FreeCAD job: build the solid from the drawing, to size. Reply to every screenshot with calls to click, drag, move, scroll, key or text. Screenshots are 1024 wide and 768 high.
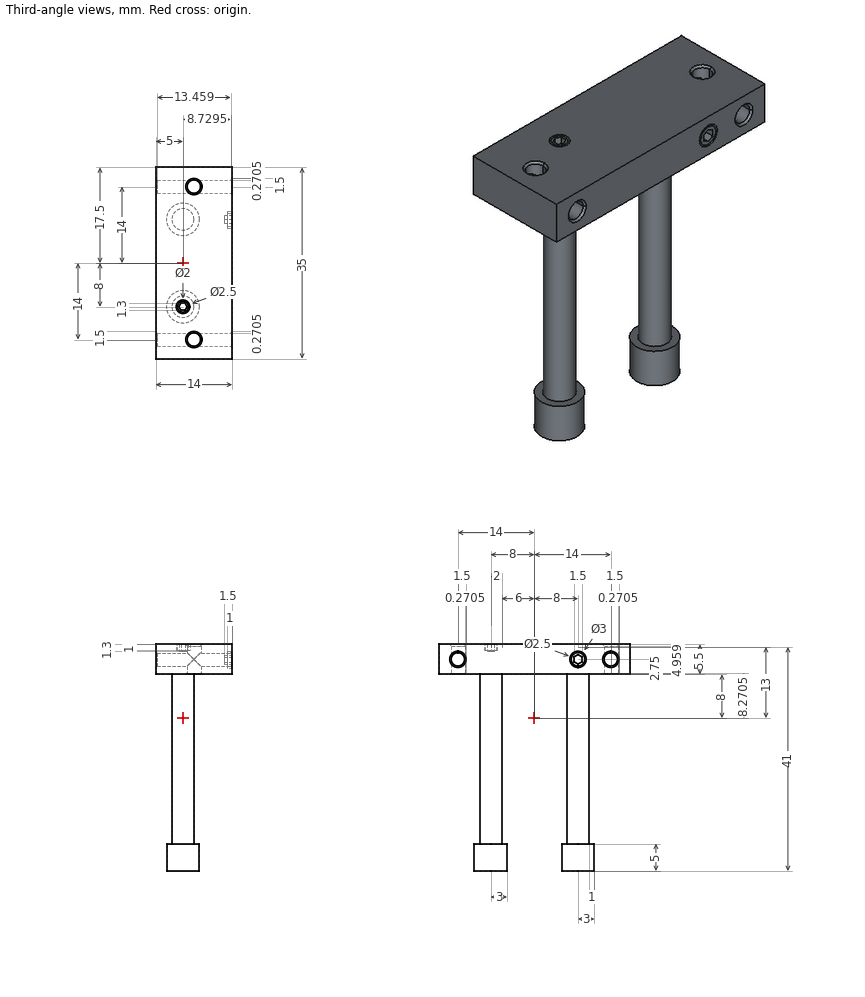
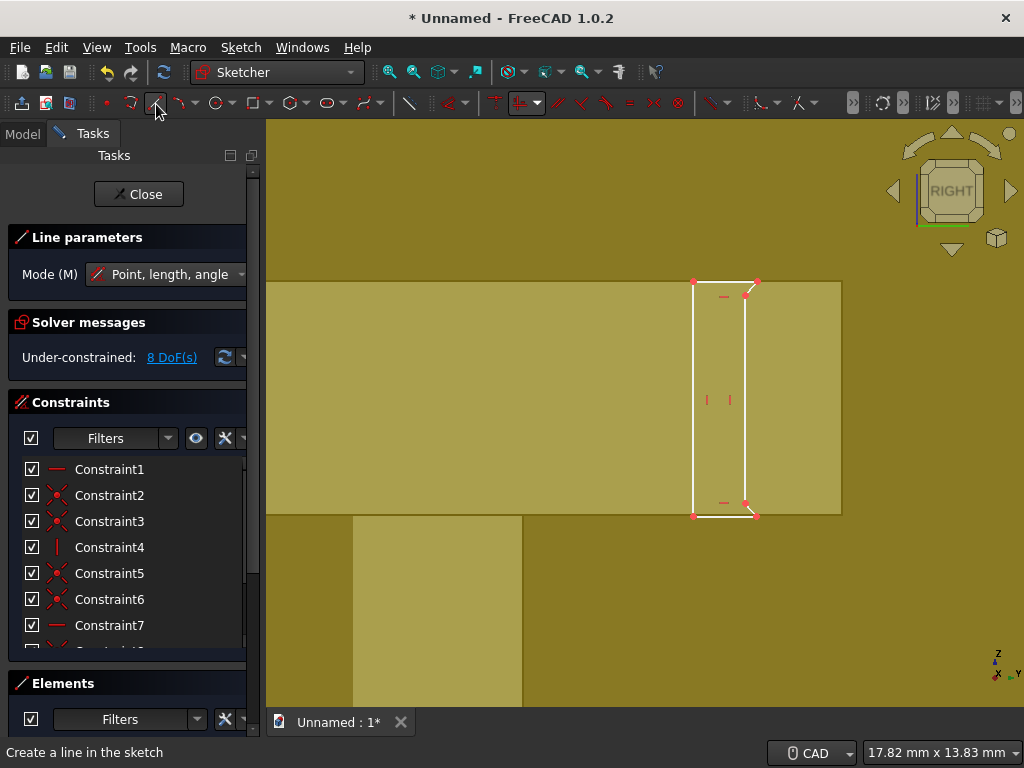
click(693, 258)
click(693, 188)
key(Escape)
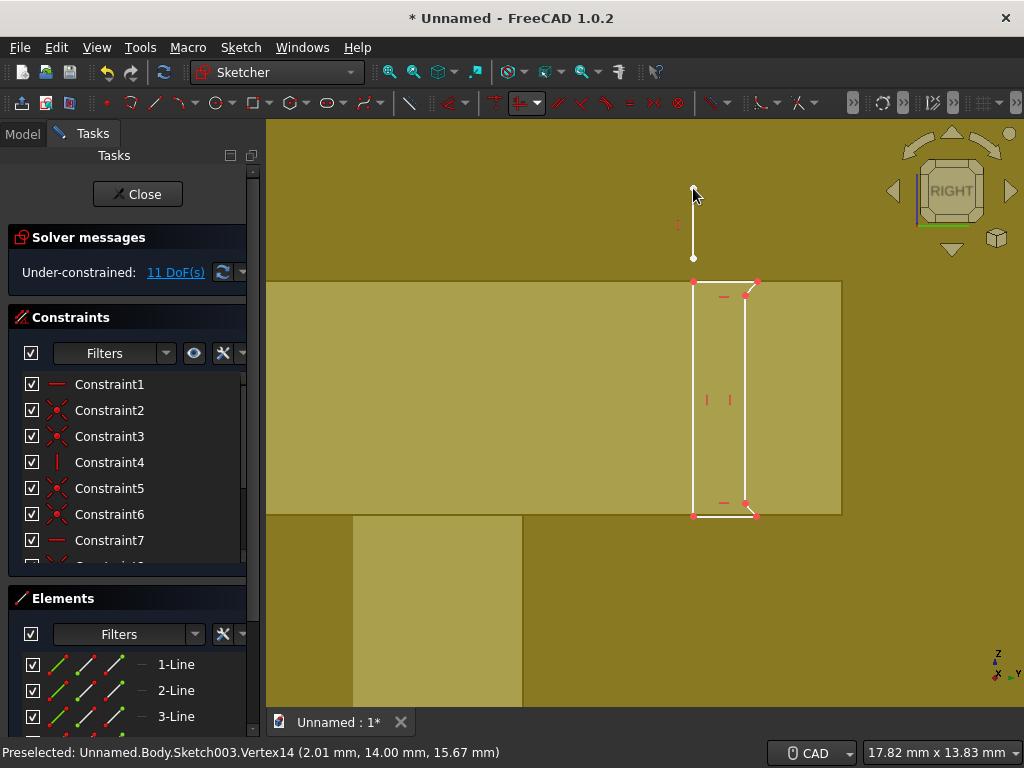
click(693, 238)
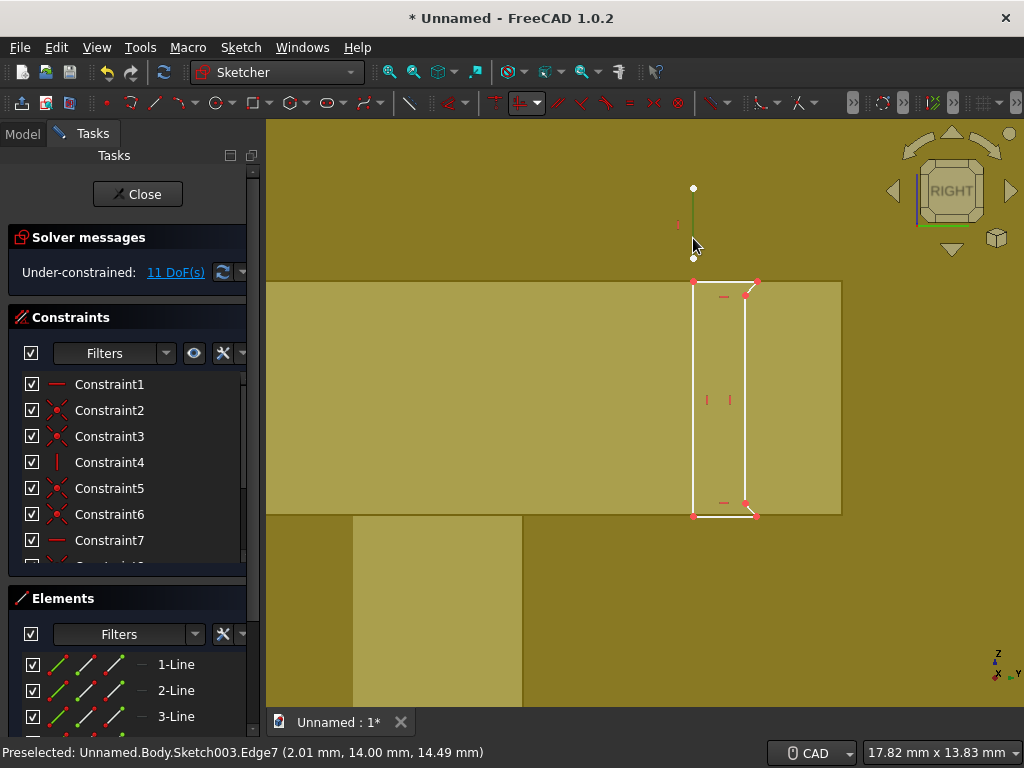
click(410, 104)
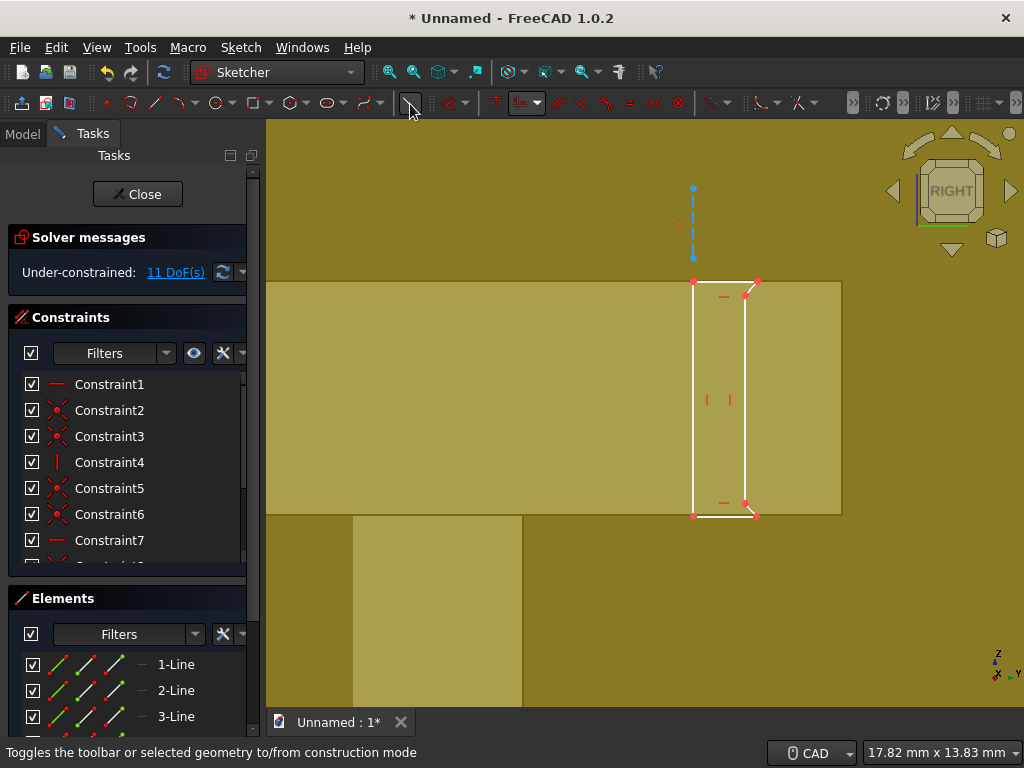
click(448, 104)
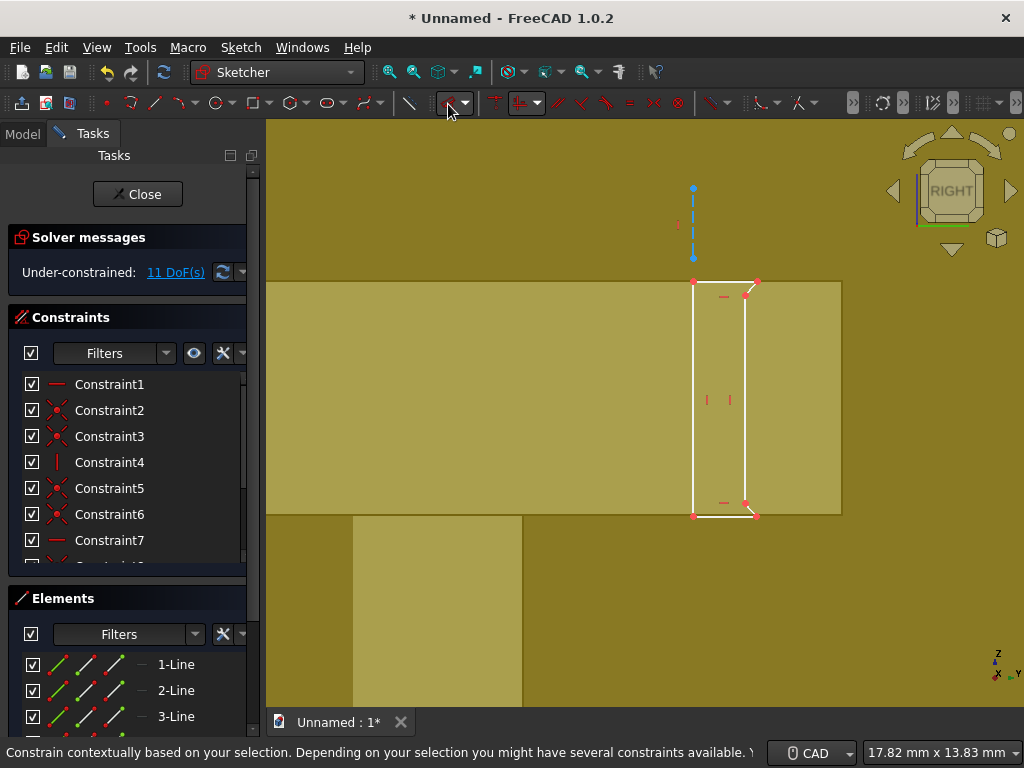
click(693, 517)
click(727, 598)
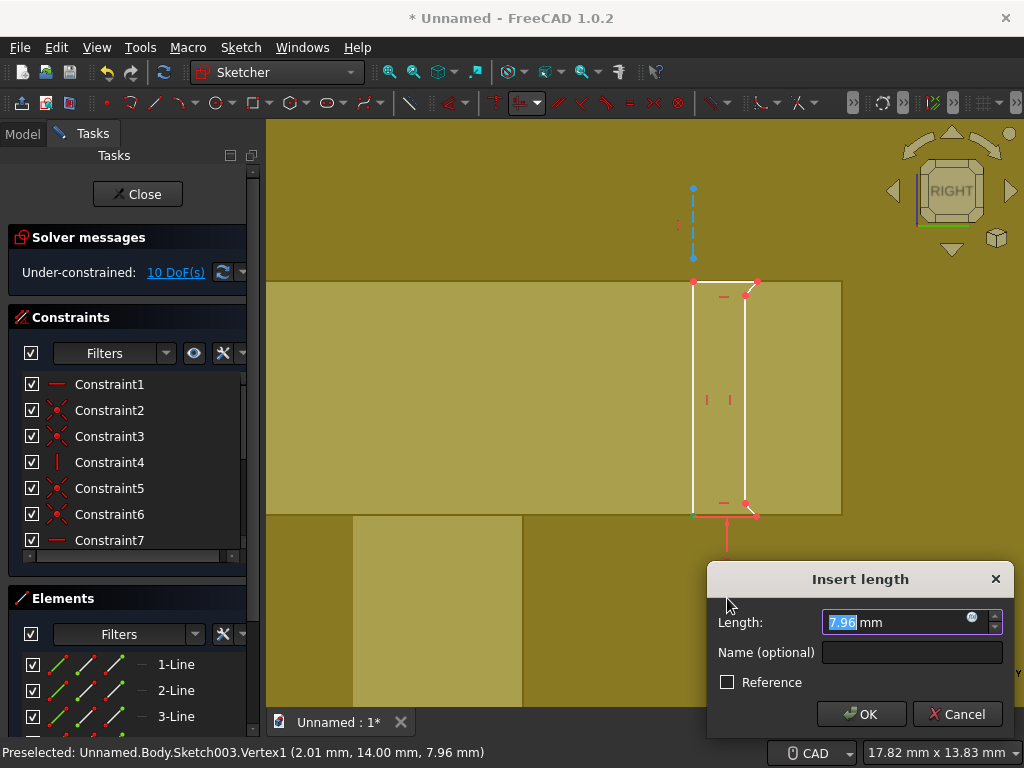
text(8)
key(Return)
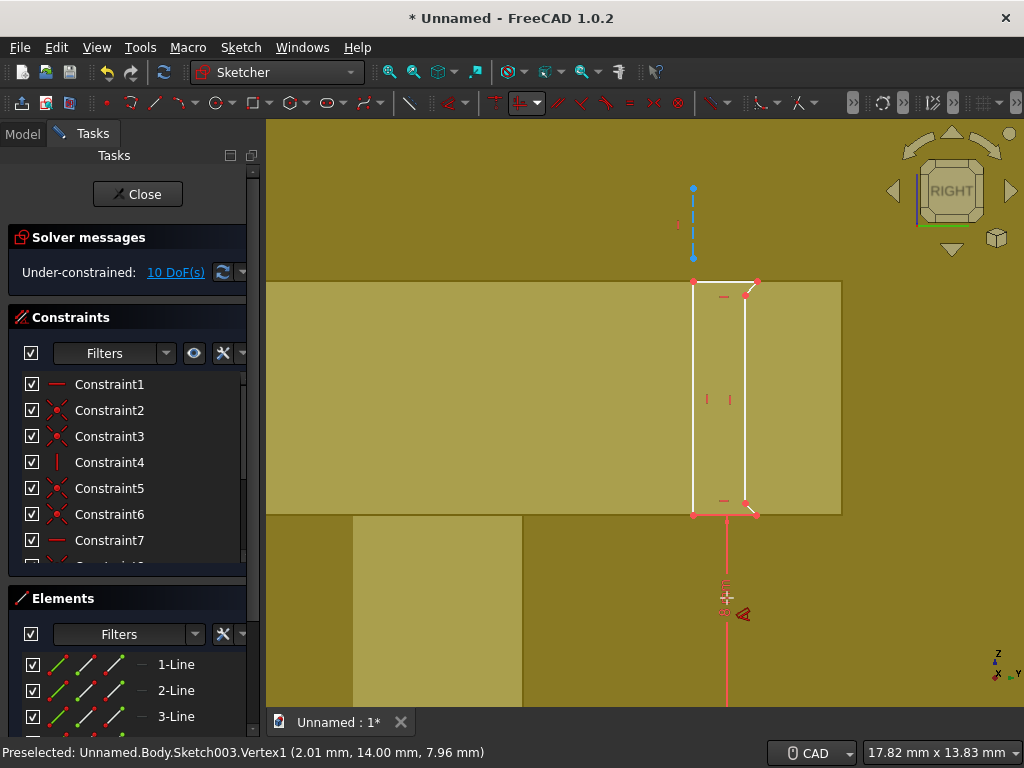
click(712, 515)
click(725, 481)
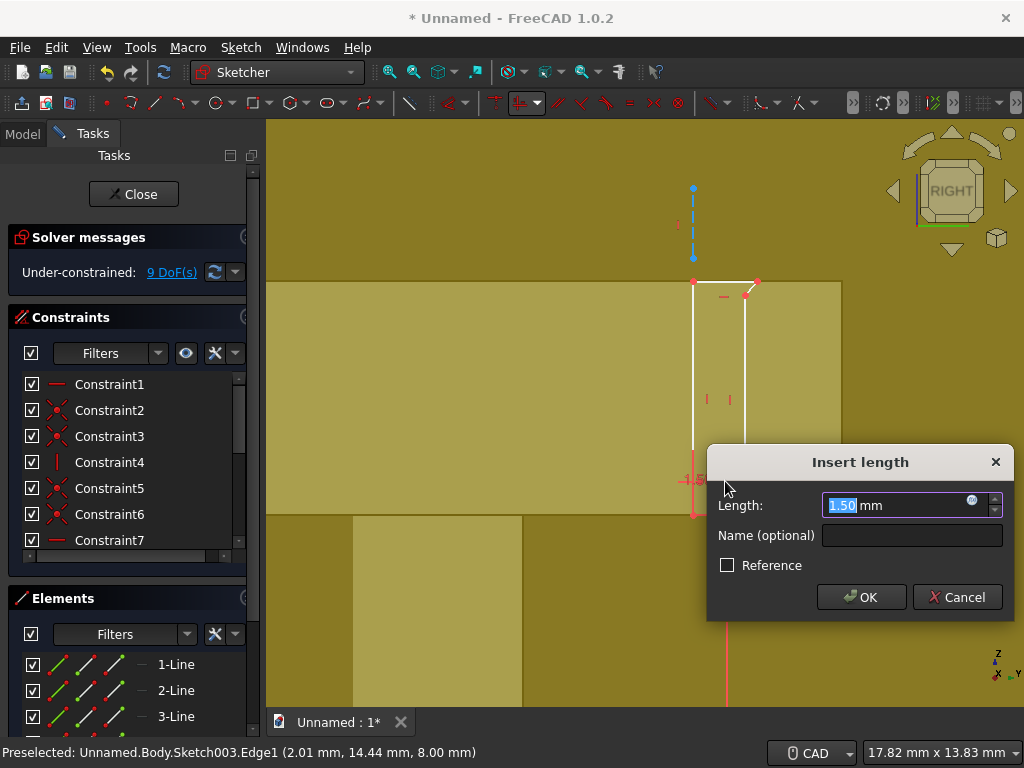
text(1.5)
key(Return)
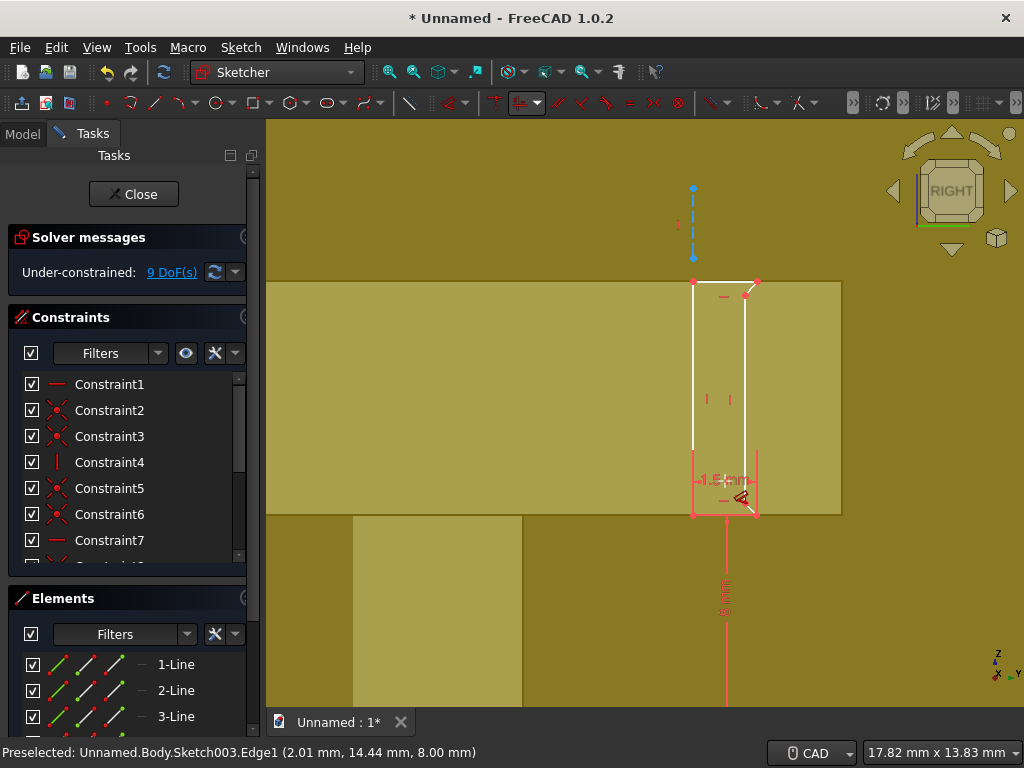
click(738, 282)
click(725, 248)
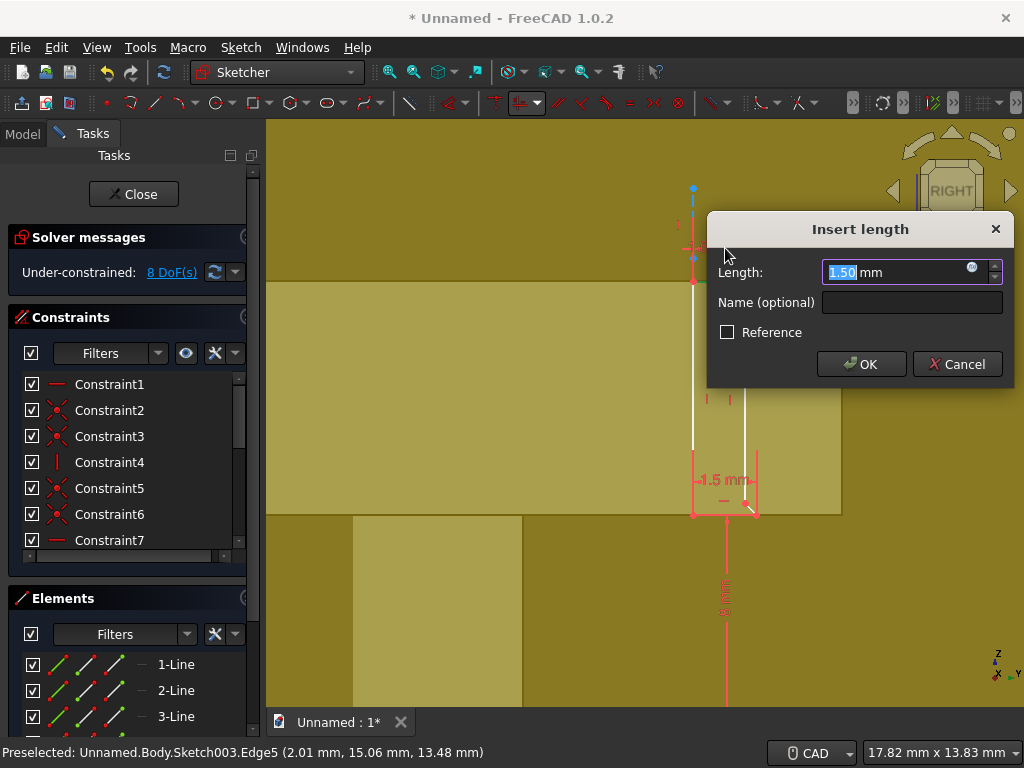
text(1.5)
key(Return)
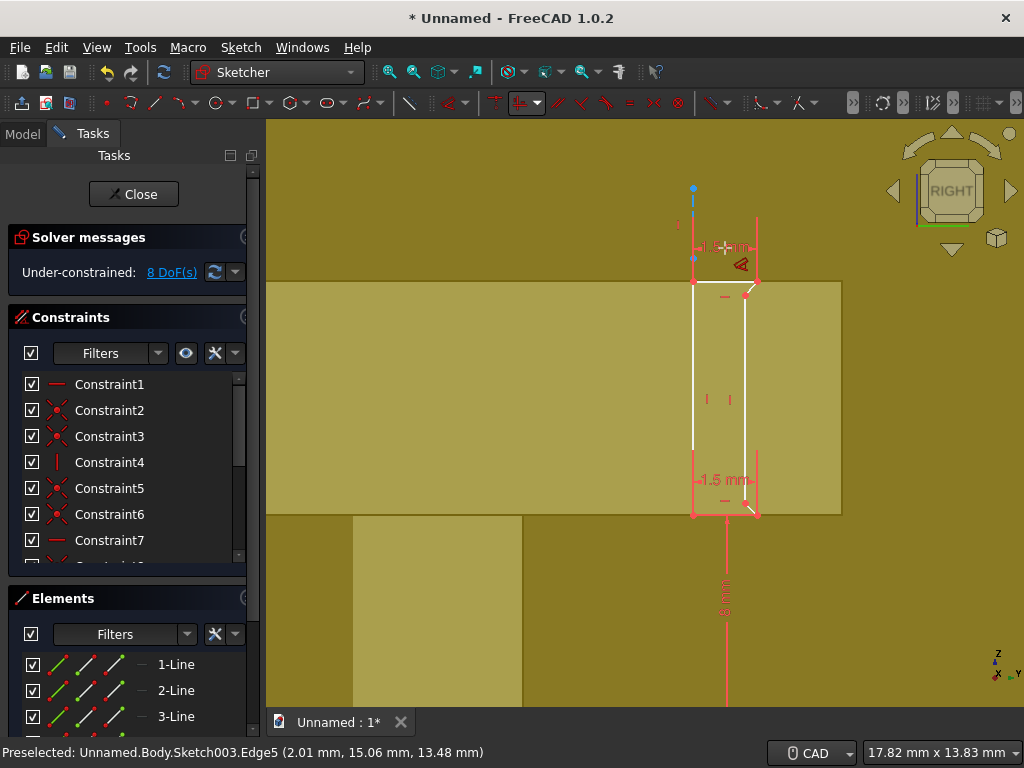
click(693, 352)
click(727, 399)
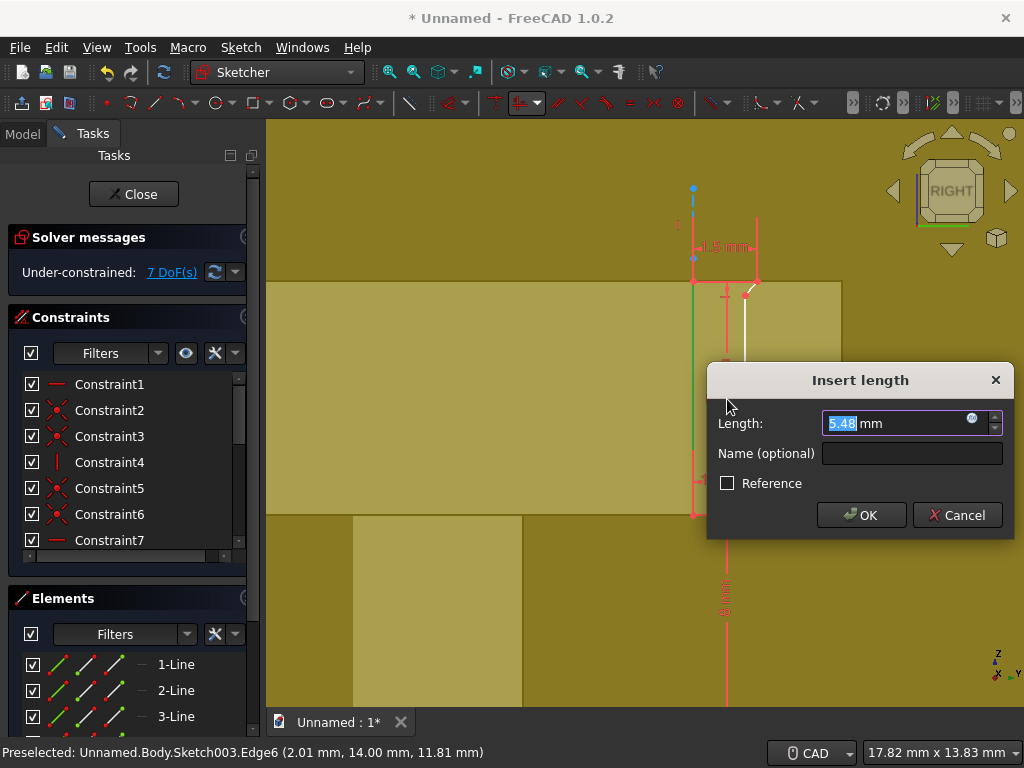
text(5.5)
key(Return)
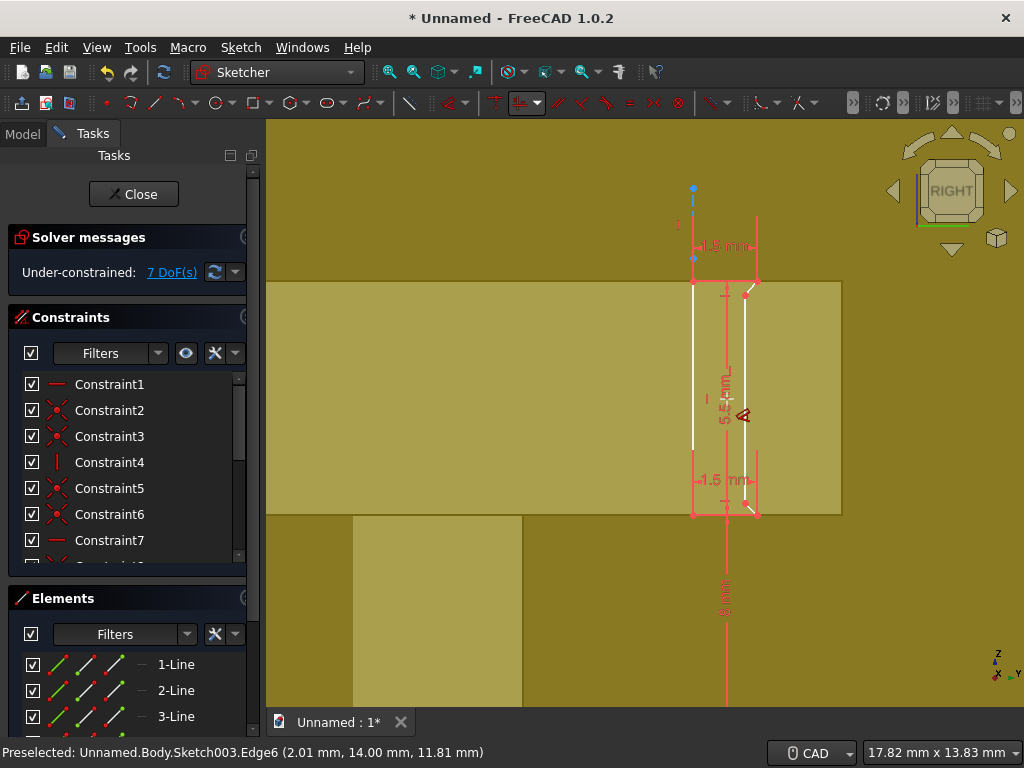
click(693, 515)
click(494, 481)